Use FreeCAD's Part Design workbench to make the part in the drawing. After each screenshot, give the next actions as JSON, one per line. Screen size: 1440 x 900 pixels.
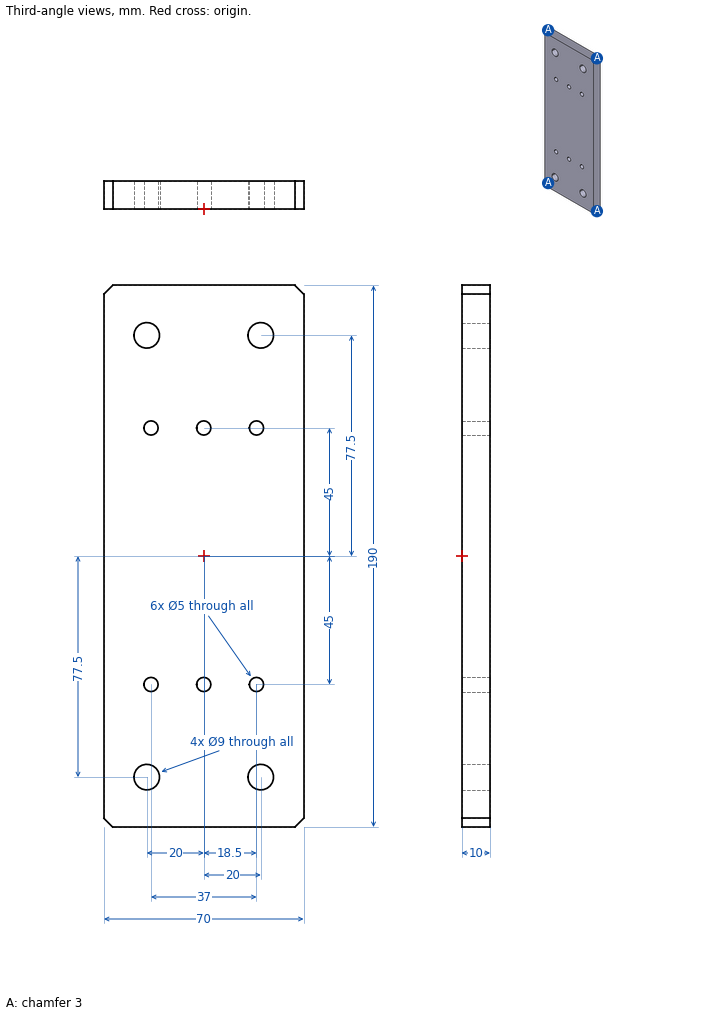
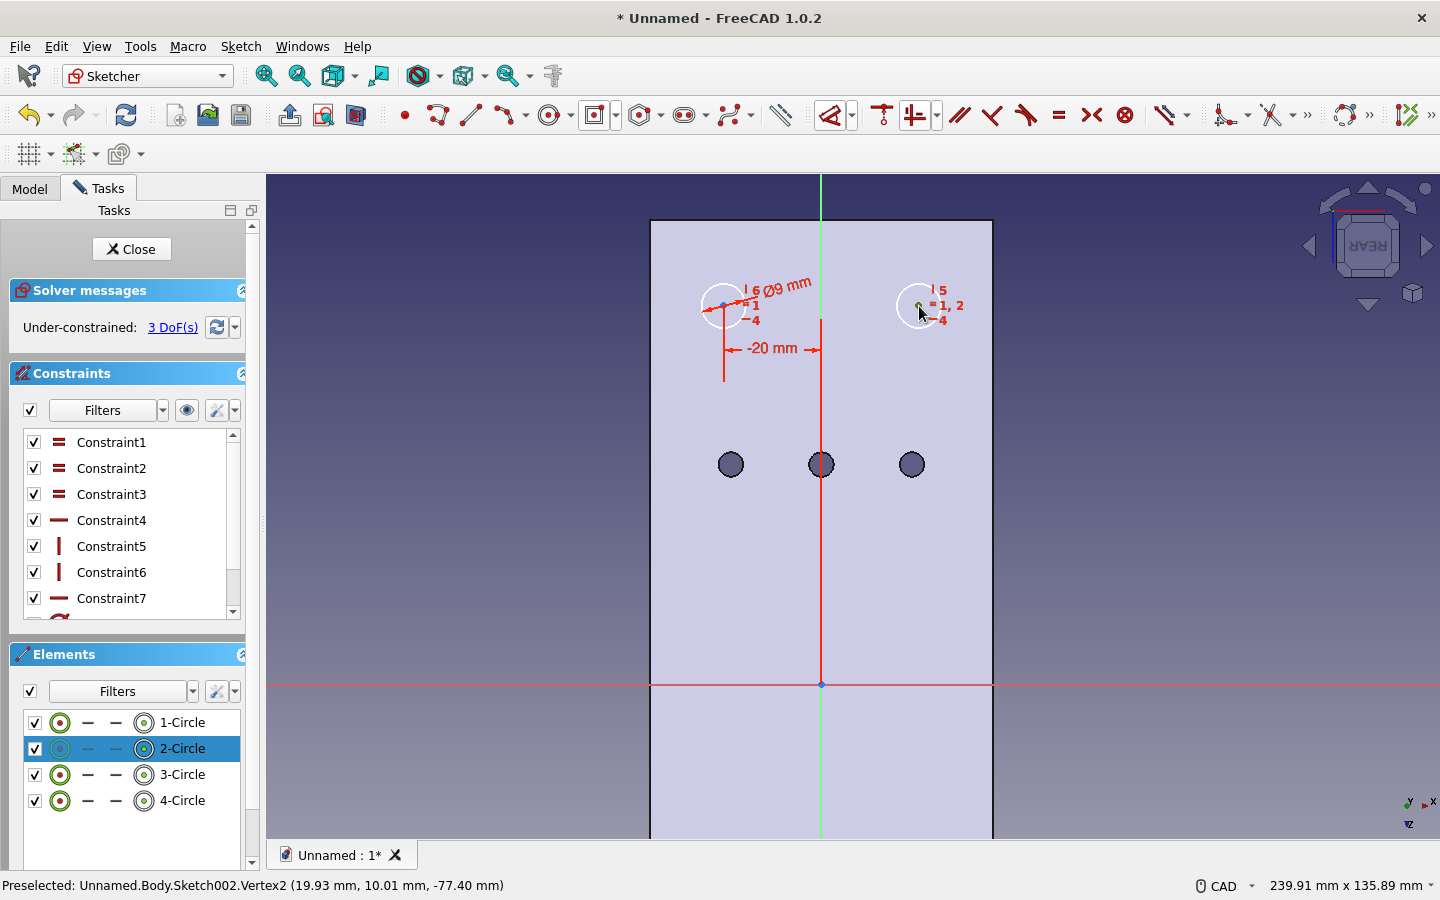
{"action": "key", "text": "l"}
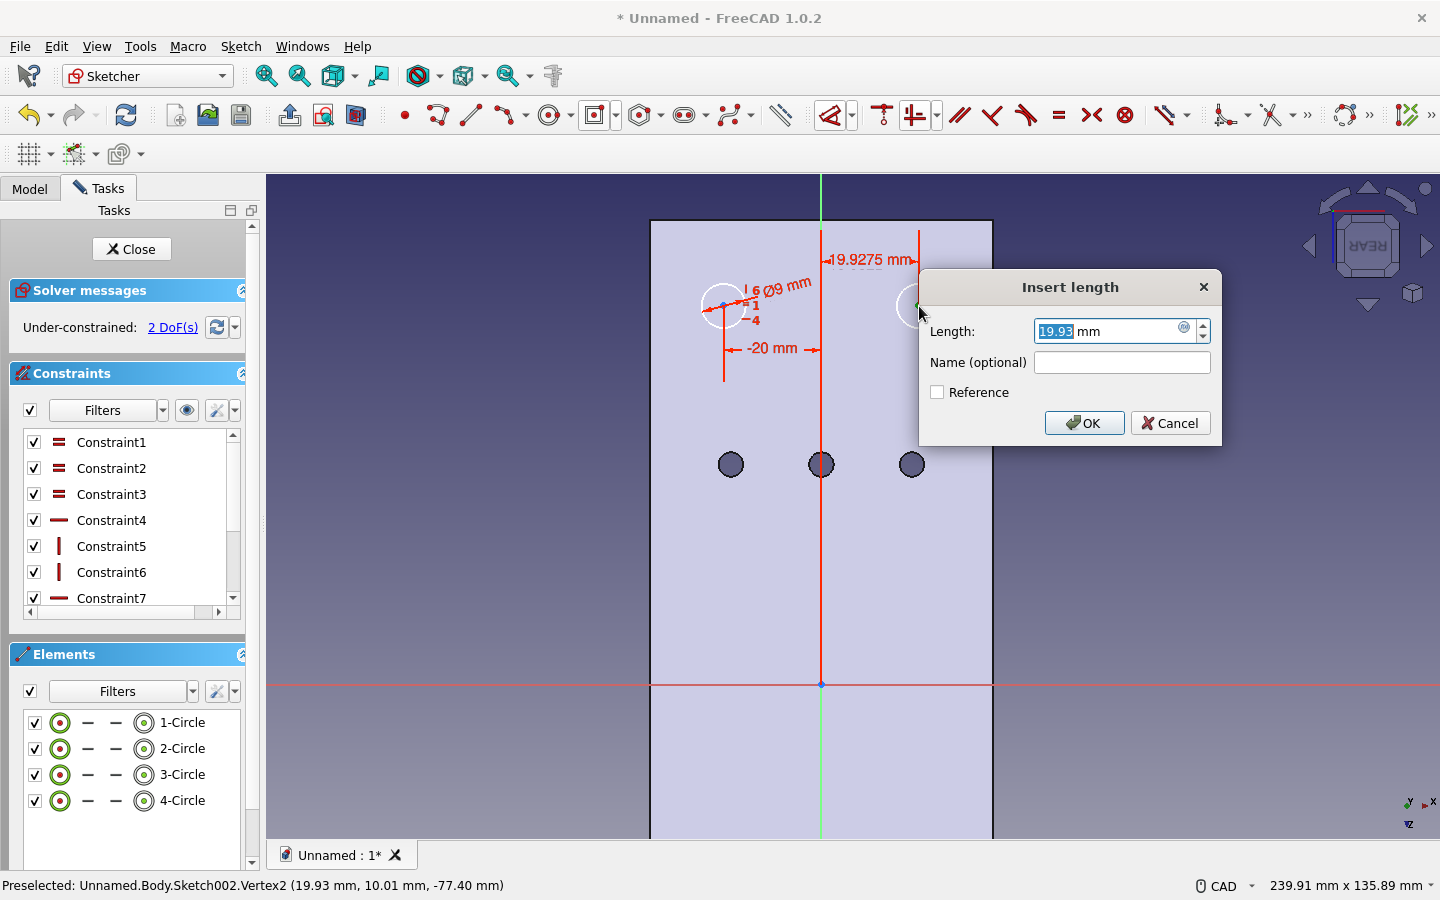
{"action": "type", "text": "20"}
{"action": "key", "text": "Return"}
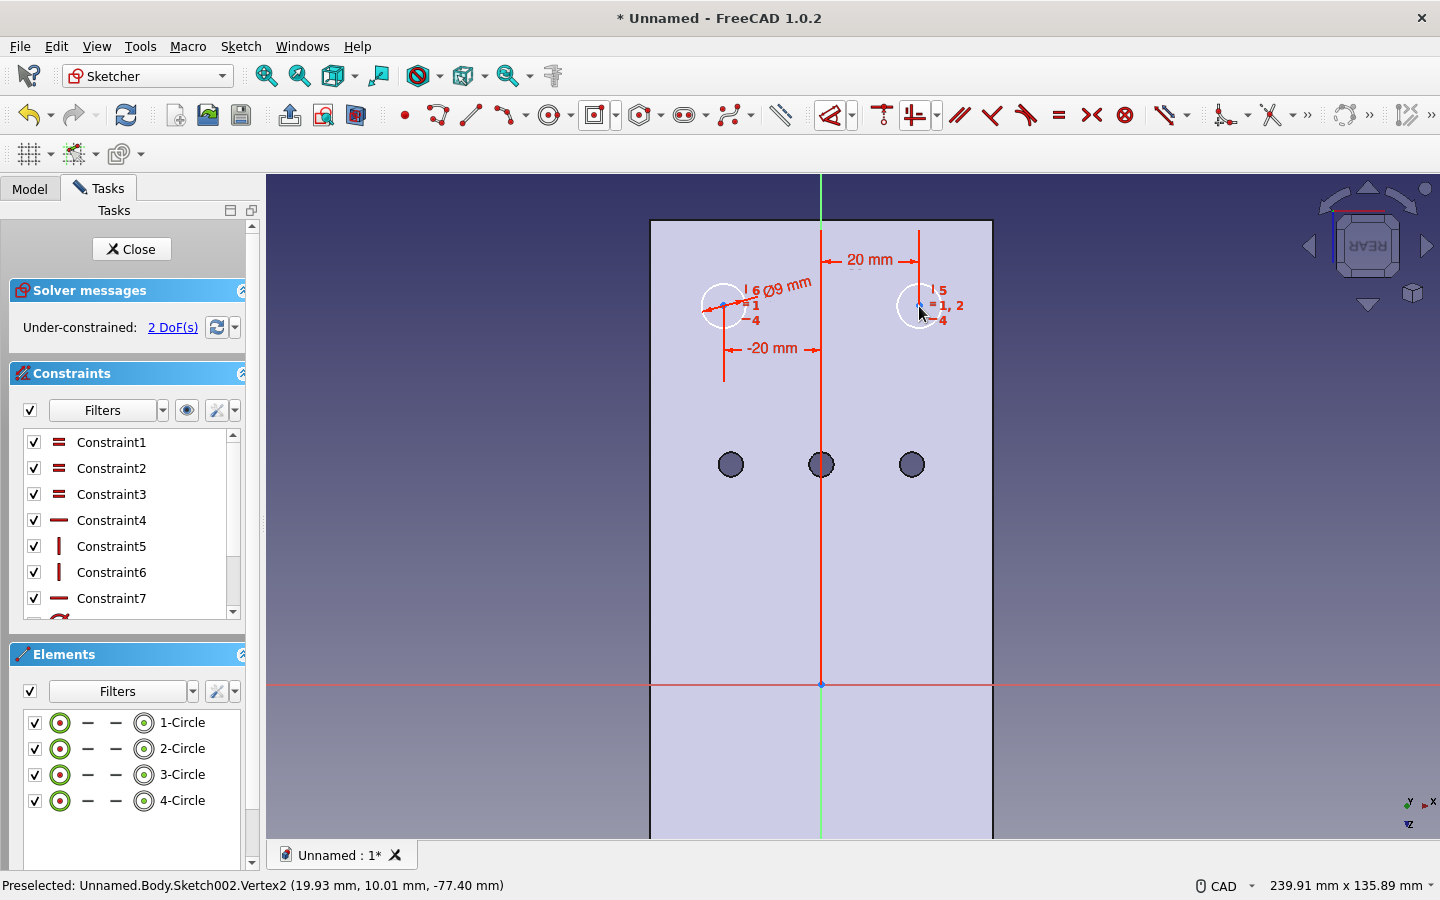
{"action": "left_click", "coordinate": [724, 306]}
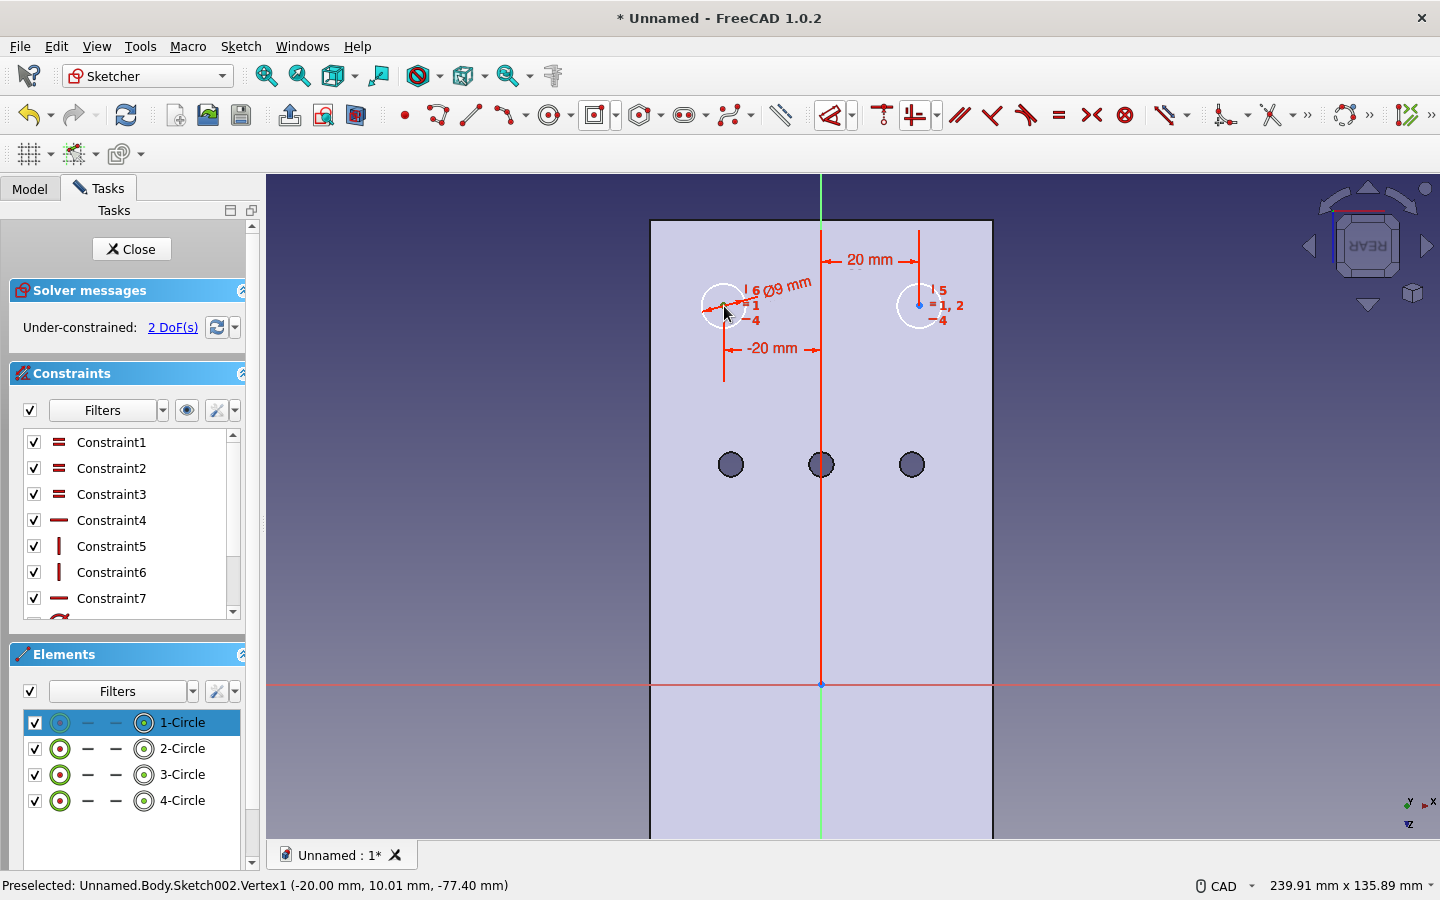
{"action": "left_click", "coordinate": [852, 116]}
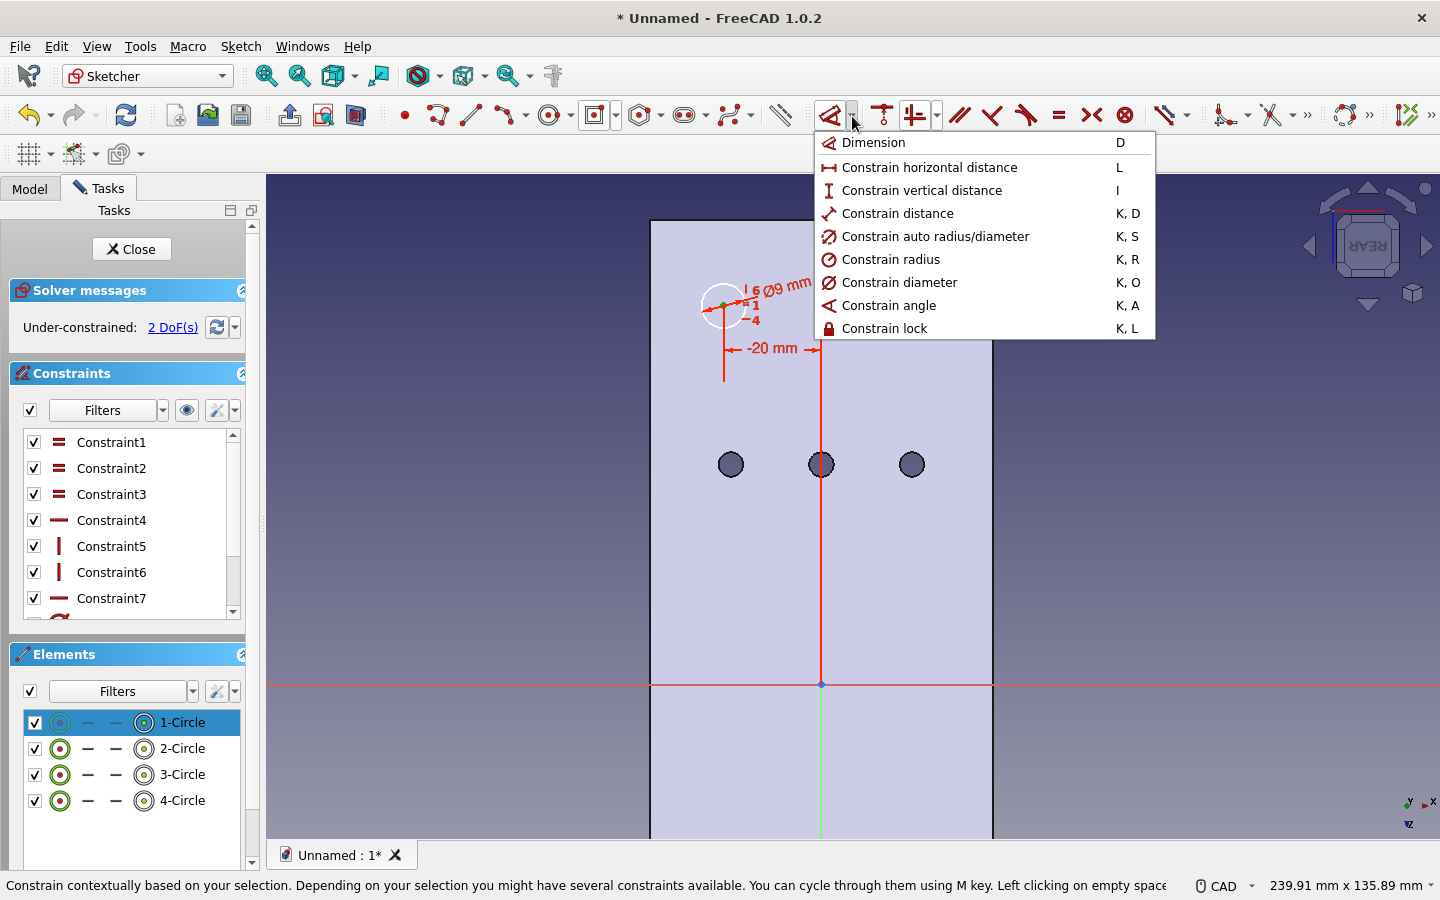
{"action": "left_click", "coordinate": [985, 190]}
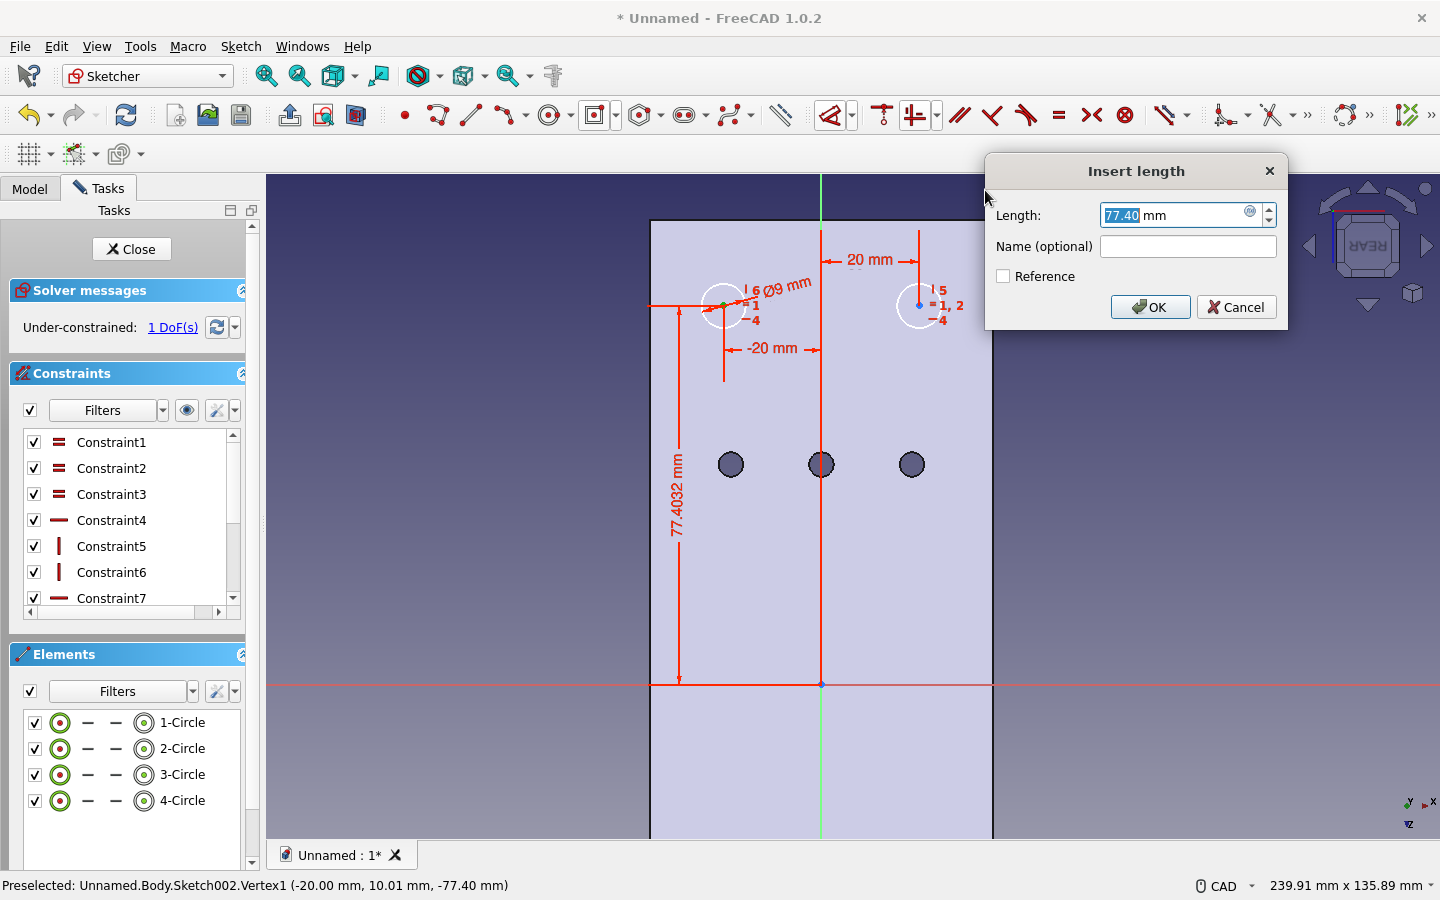
{"action": "type", "text": "77.5"}
{"action": "key", "text": "Return"}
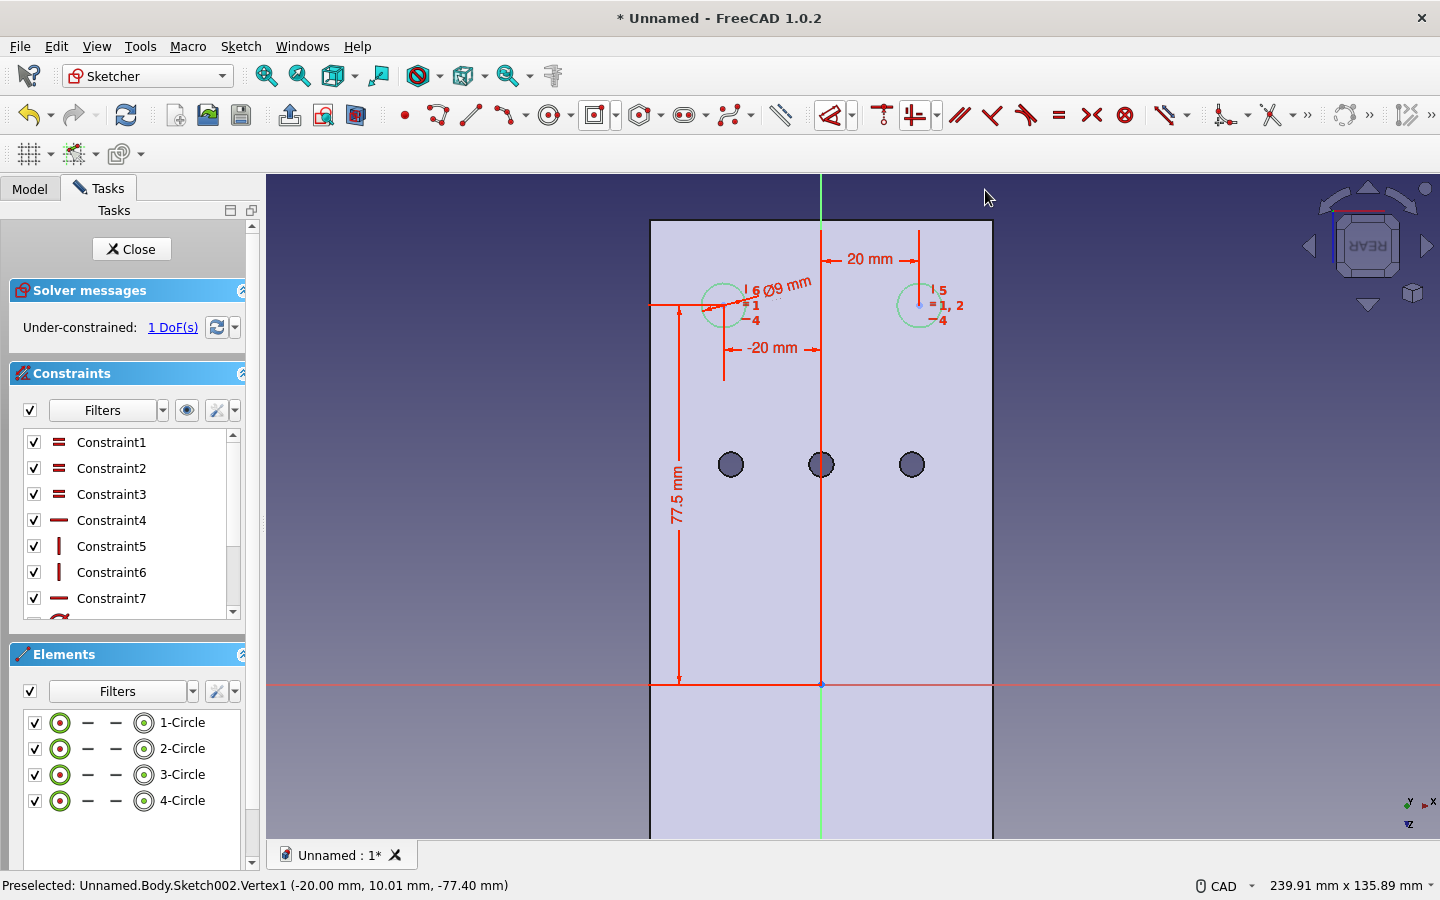
{"action": "scroll", "coordinate": [740, 290], "scroll_direction": "down", "scroll_amount": 3}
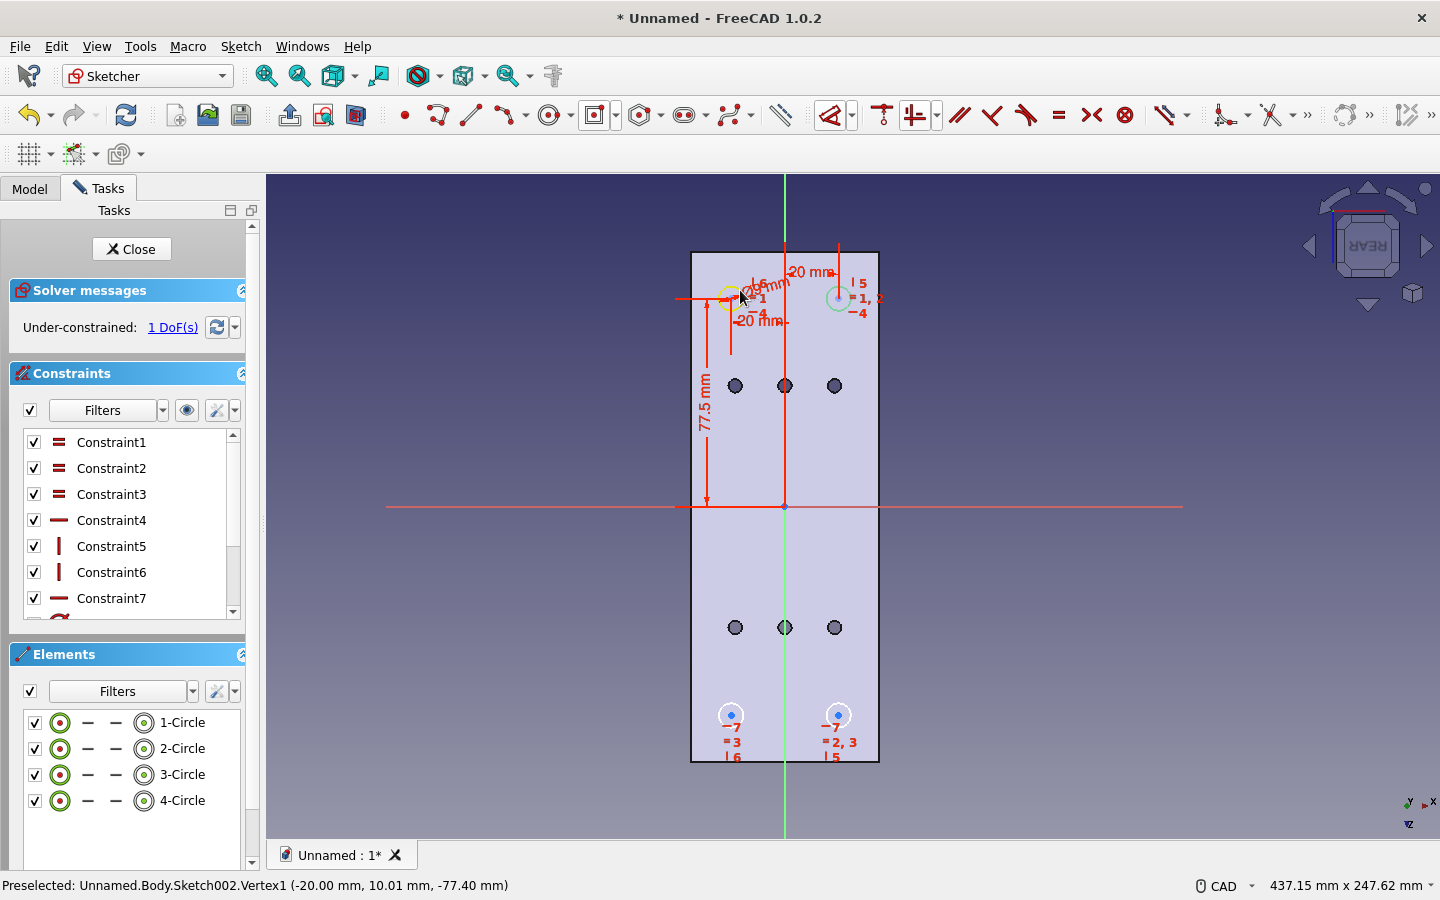
{"action": "left_click", "coordinate": [839, 715]}